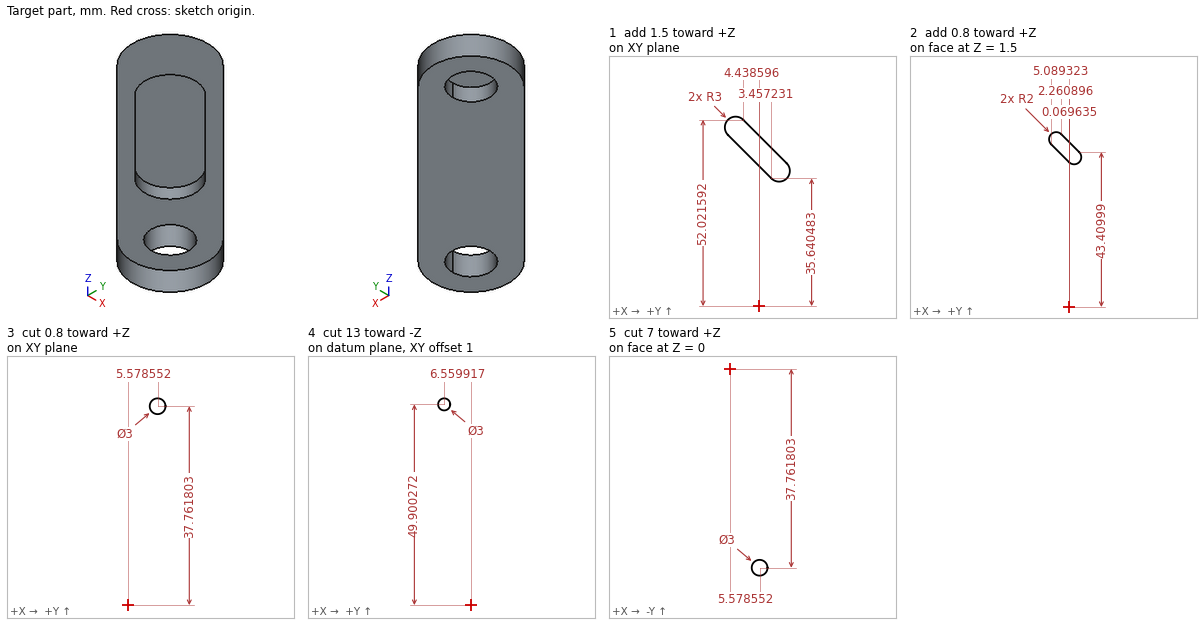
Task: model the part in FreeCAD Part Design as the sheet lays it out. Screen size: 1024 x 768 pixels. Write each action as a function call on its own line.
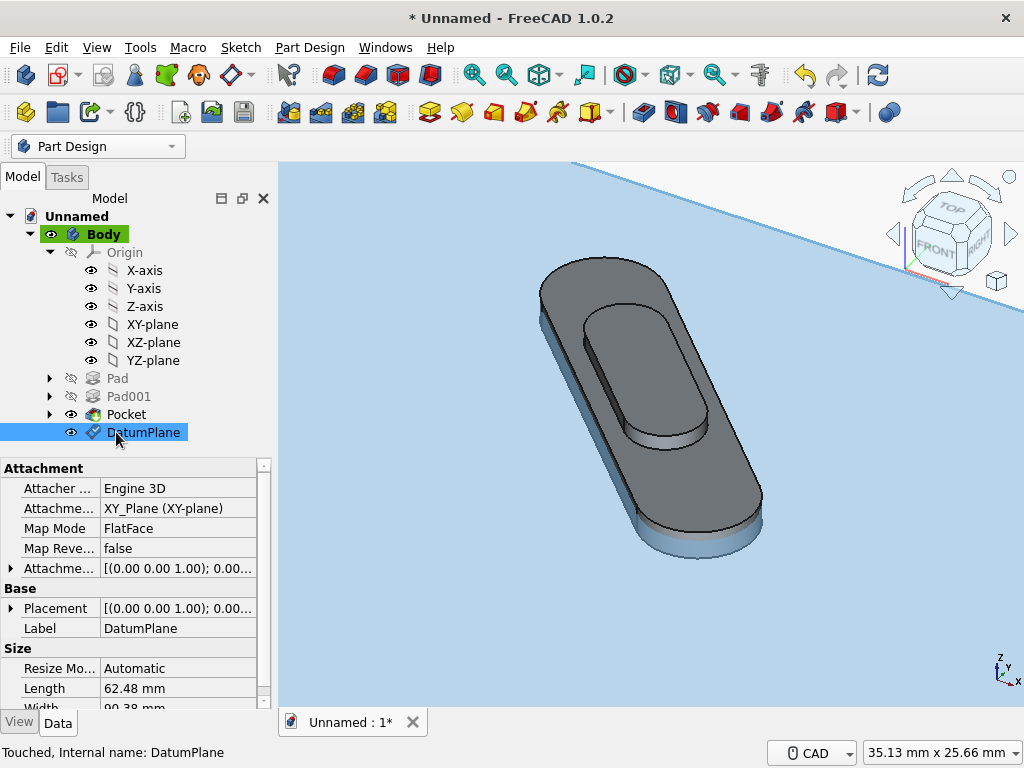
click(58, 76)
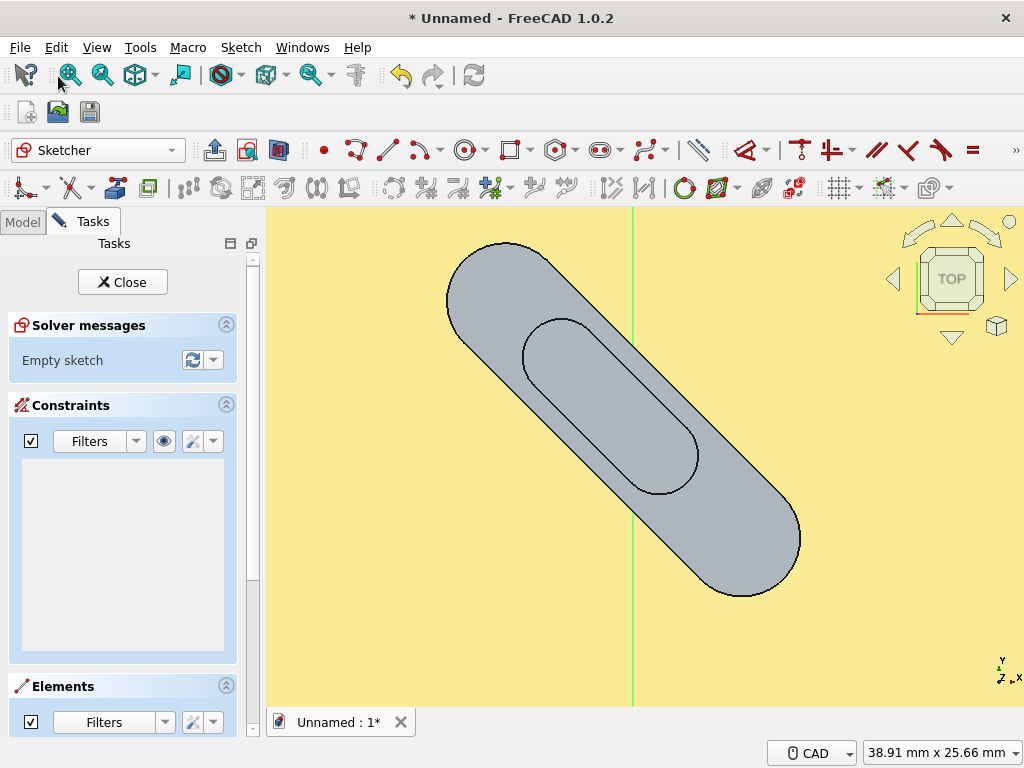
click(280, 150)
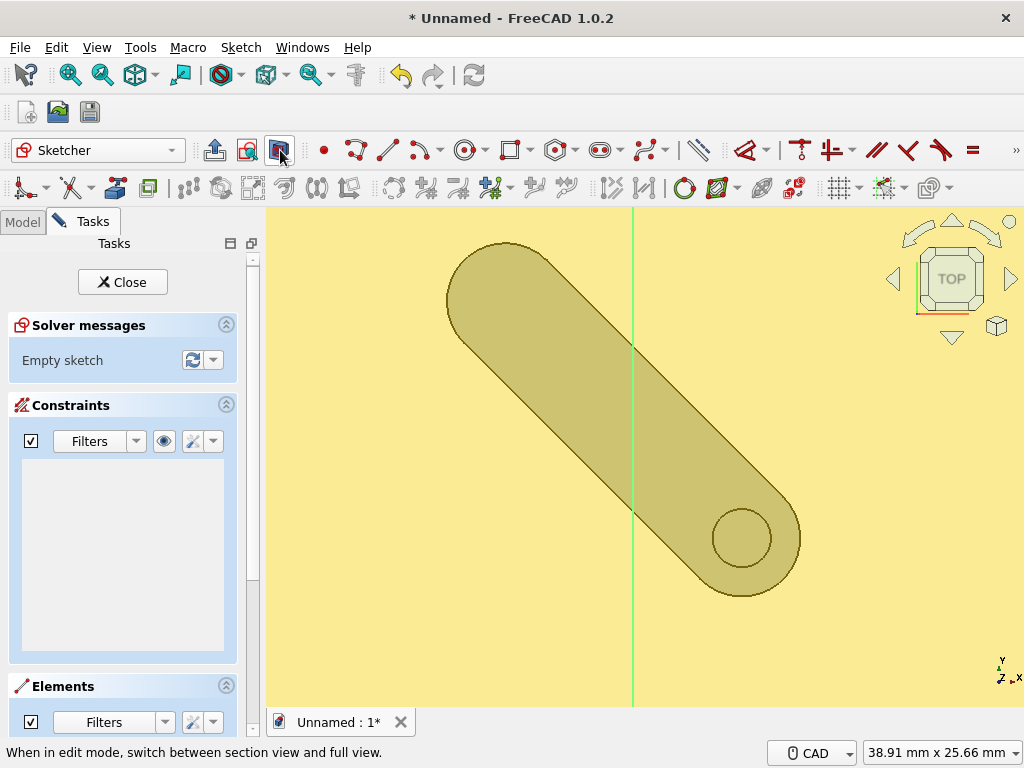
scroll(487, 262, up, 8)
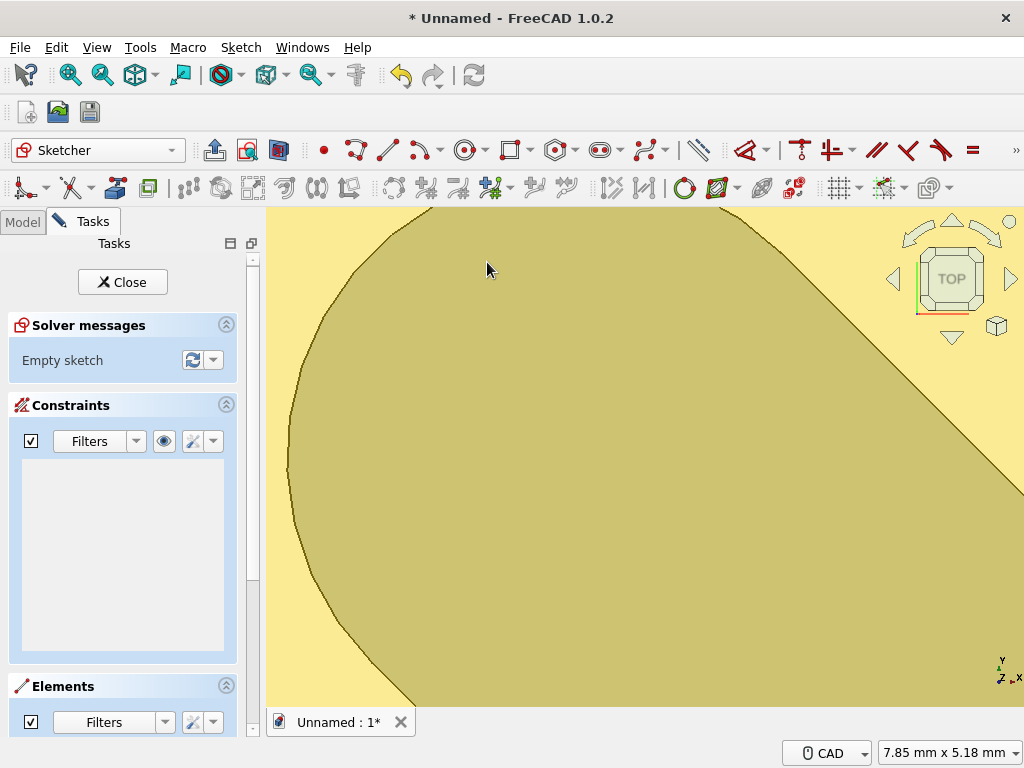
click(466, 150)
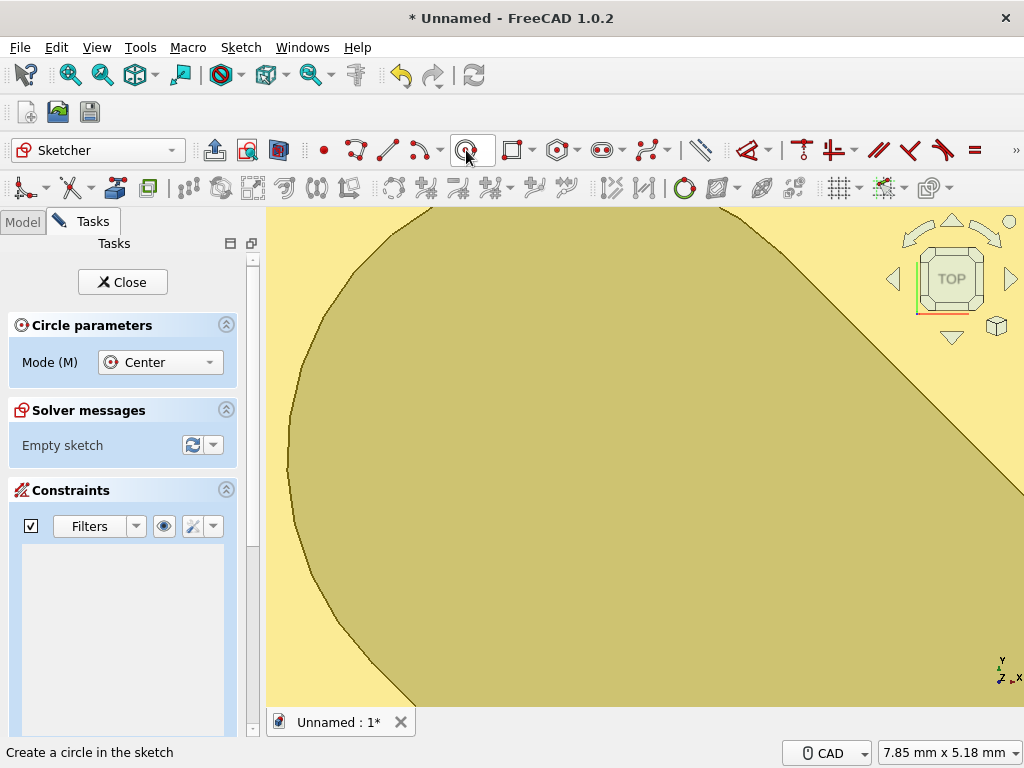
click(577, 458)
click(679, 355)
key(Escape)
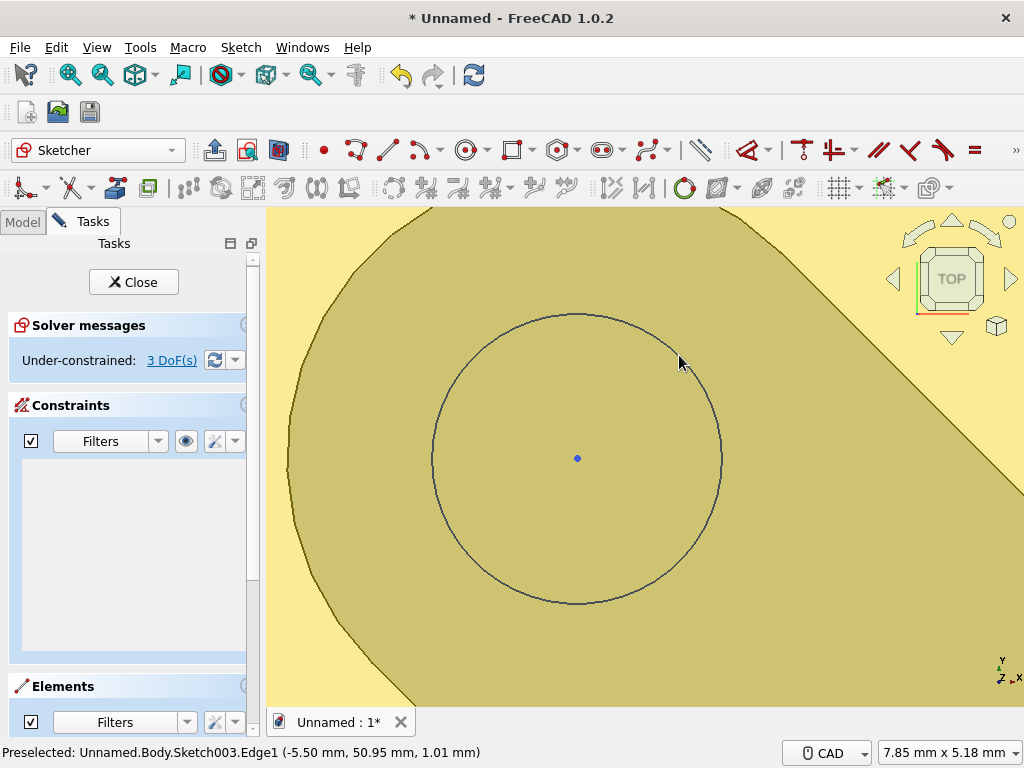
key(d)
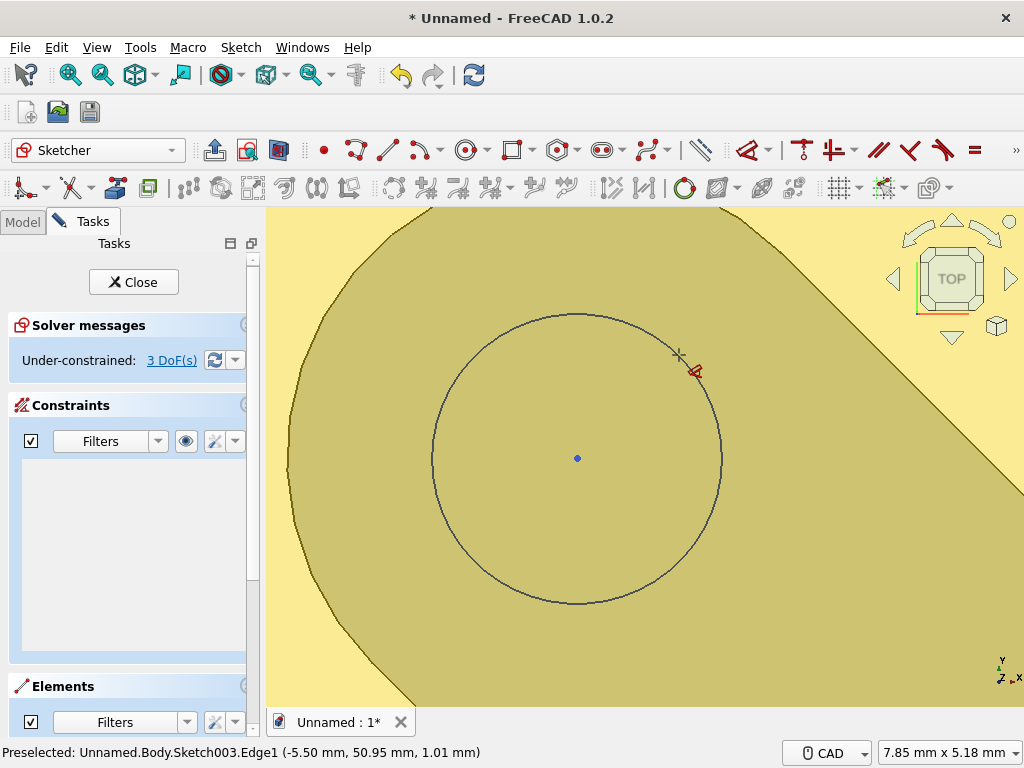
click(679, 356)
click(702, 333)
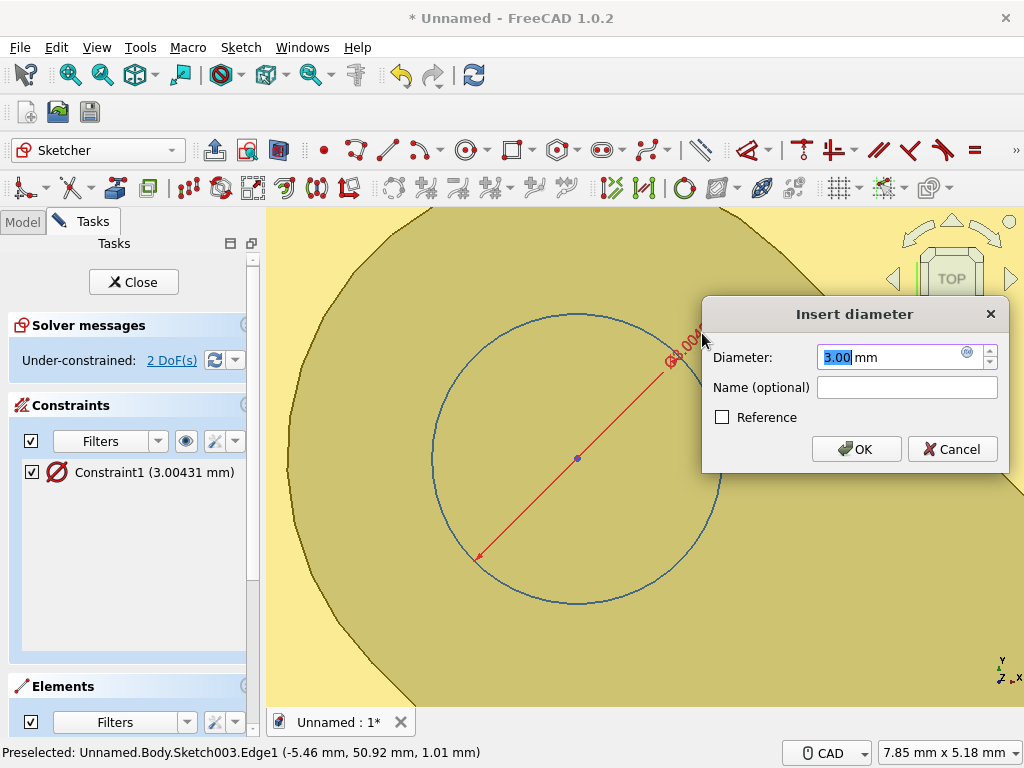
text(3)
key(Return)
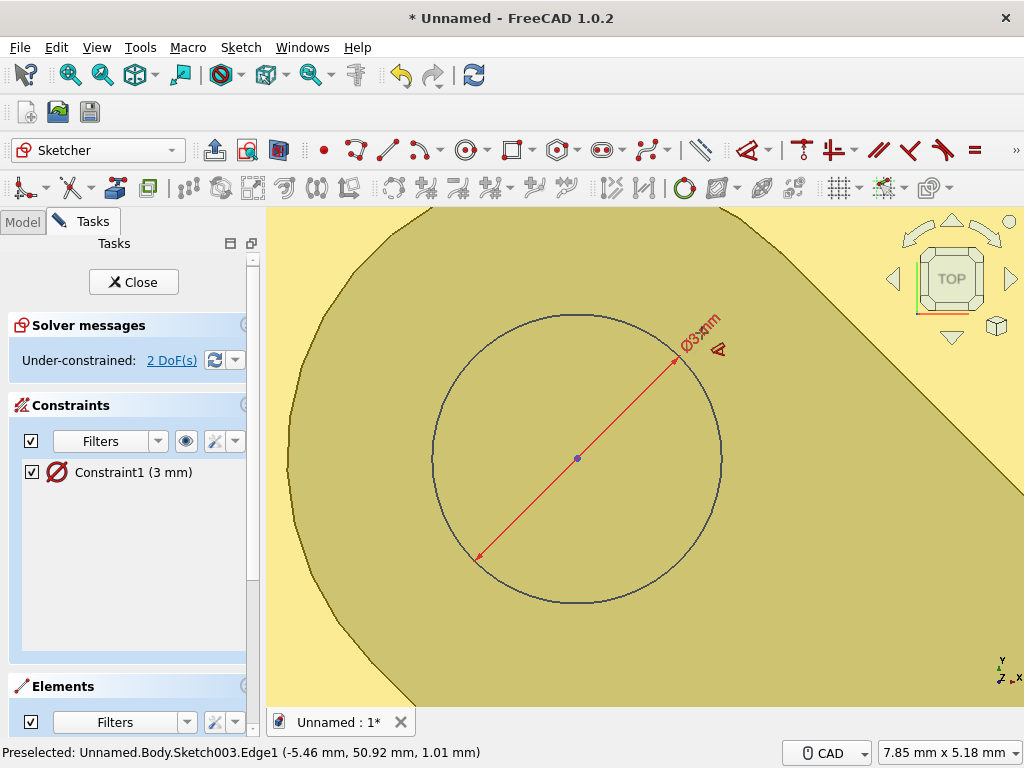
click(577, 459)
click(653, 425)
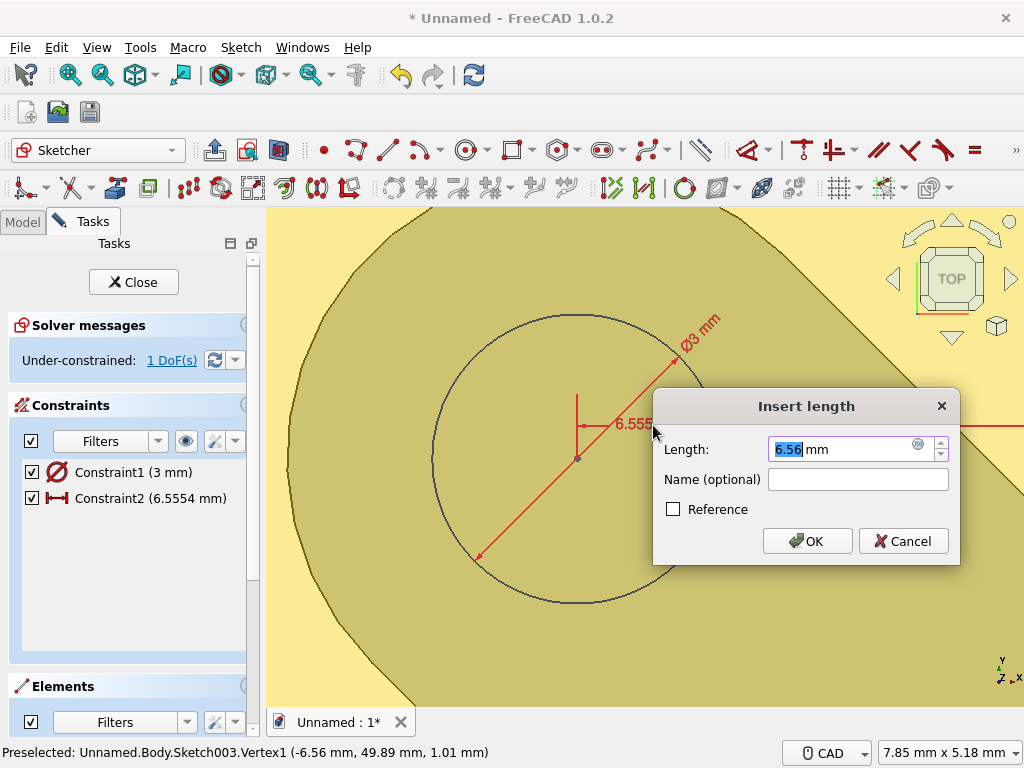
text(6.559917)
key(Return)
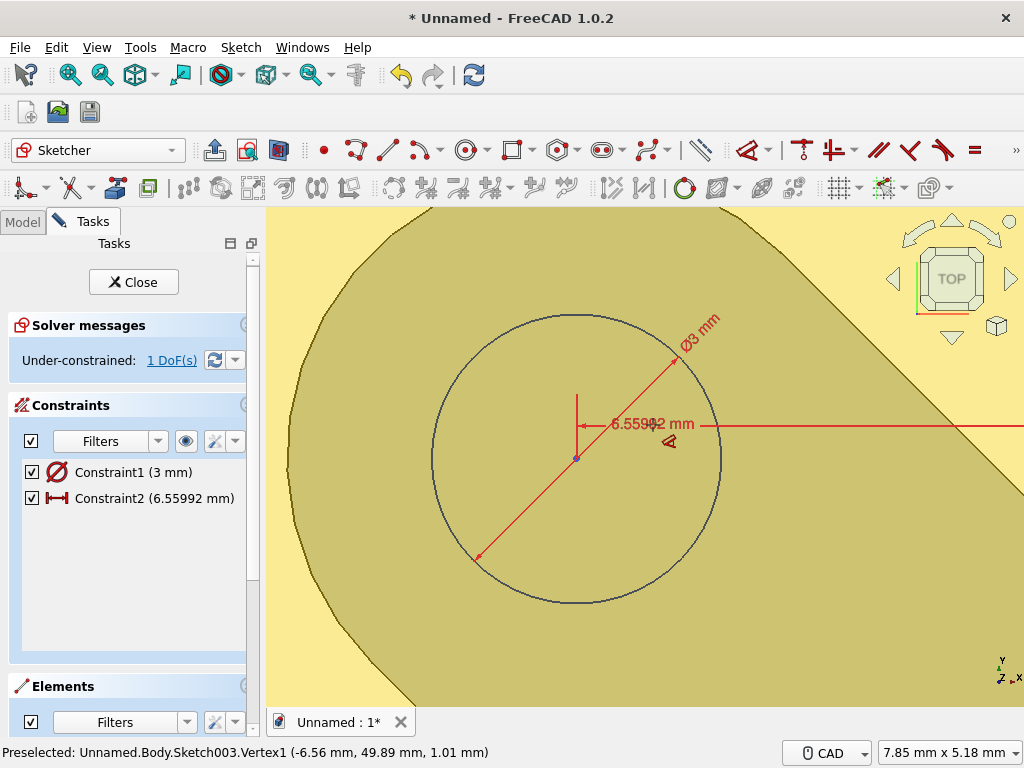
click(577, 459)
click(543, 569)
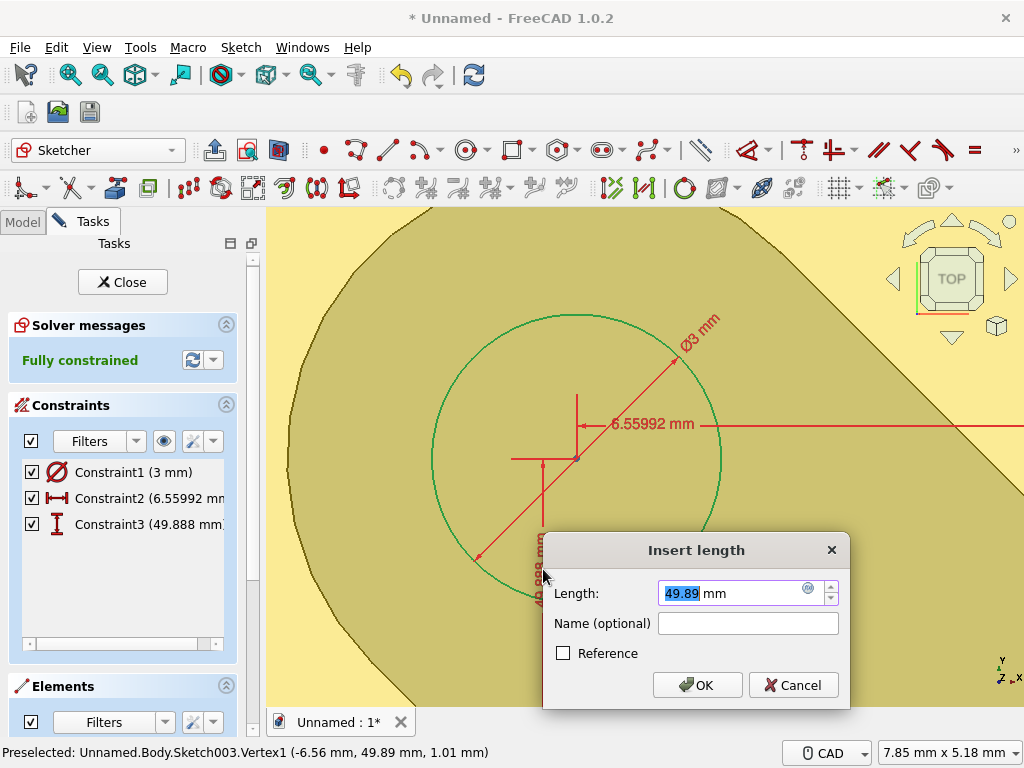
text(49.900272)
key(Return)
key(Escape)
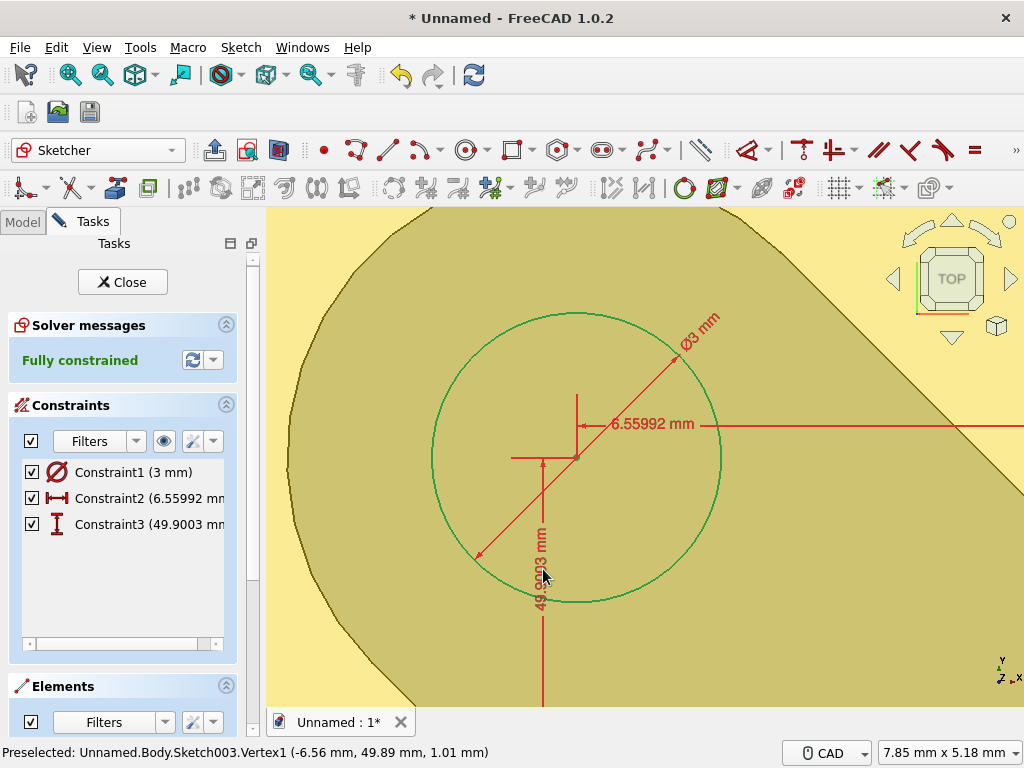
click(123, 282)